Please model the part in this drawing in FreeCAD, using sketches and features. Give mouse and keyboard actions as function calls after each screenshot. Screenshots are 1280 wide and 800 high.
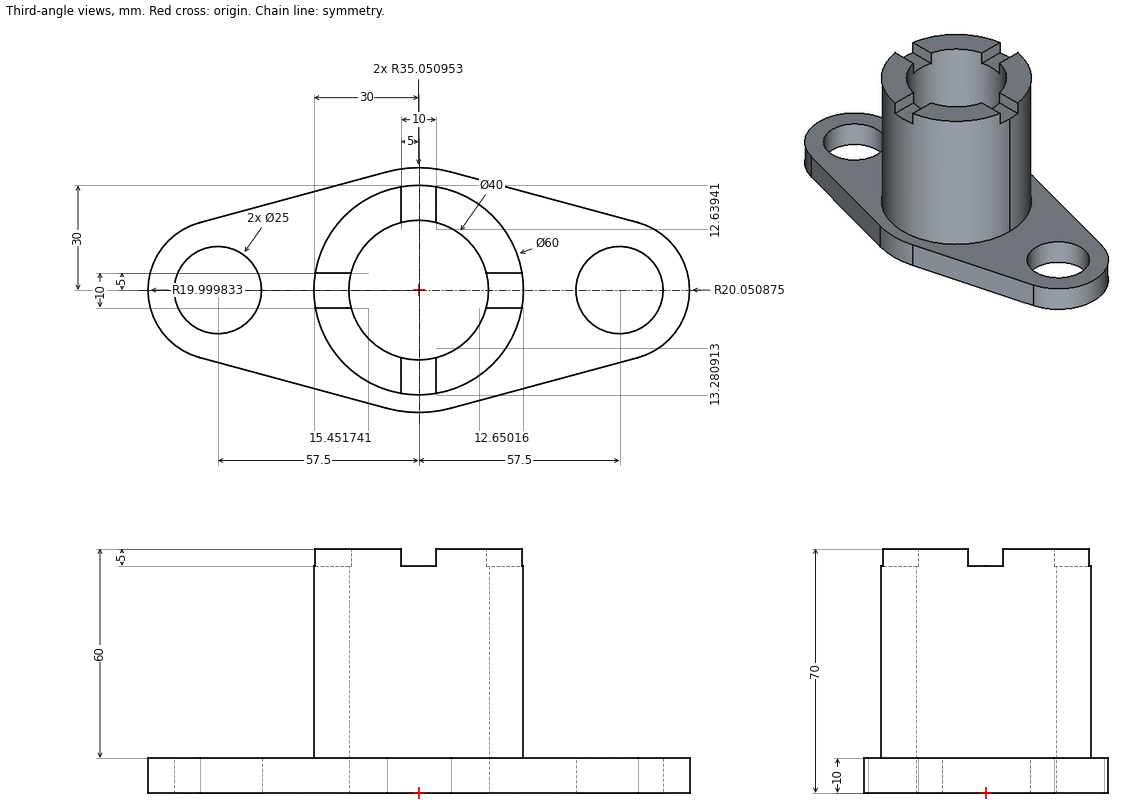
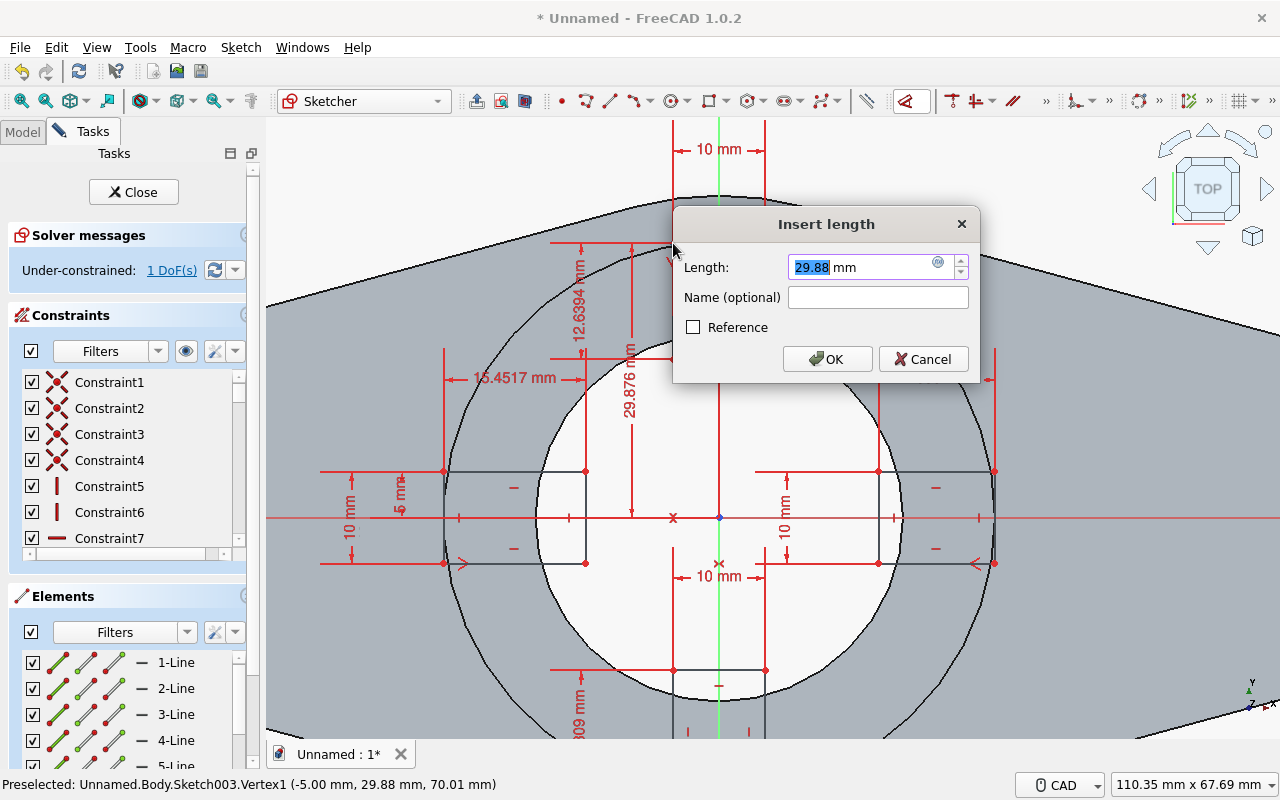
text(30)
key(Return)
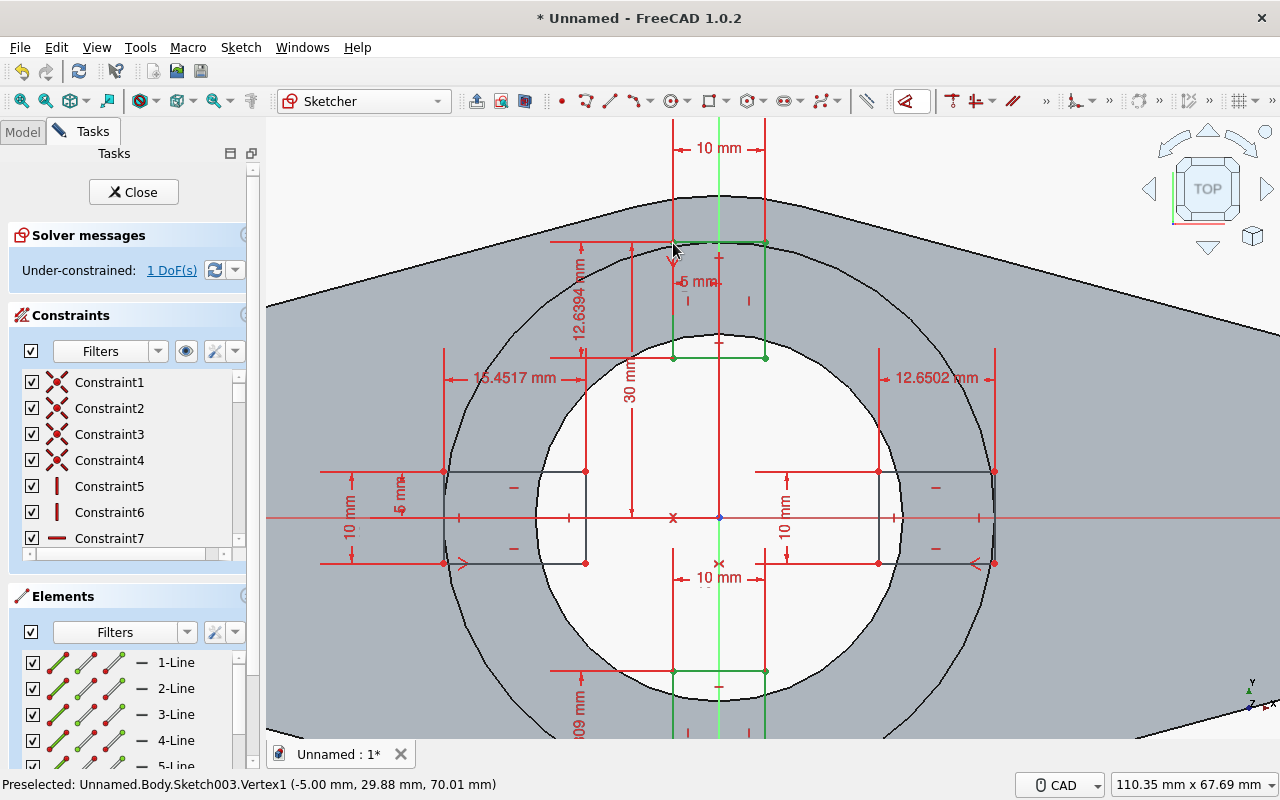
click(444, 472)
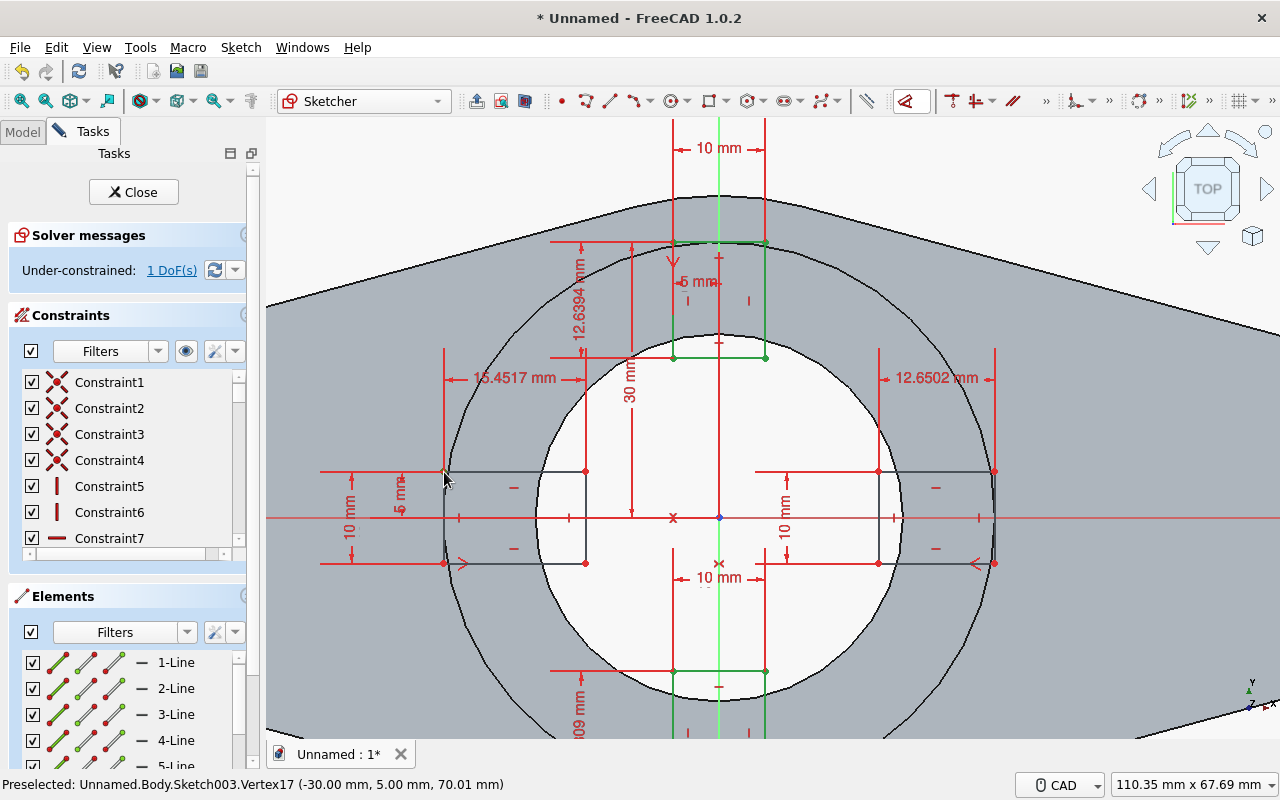
key(l)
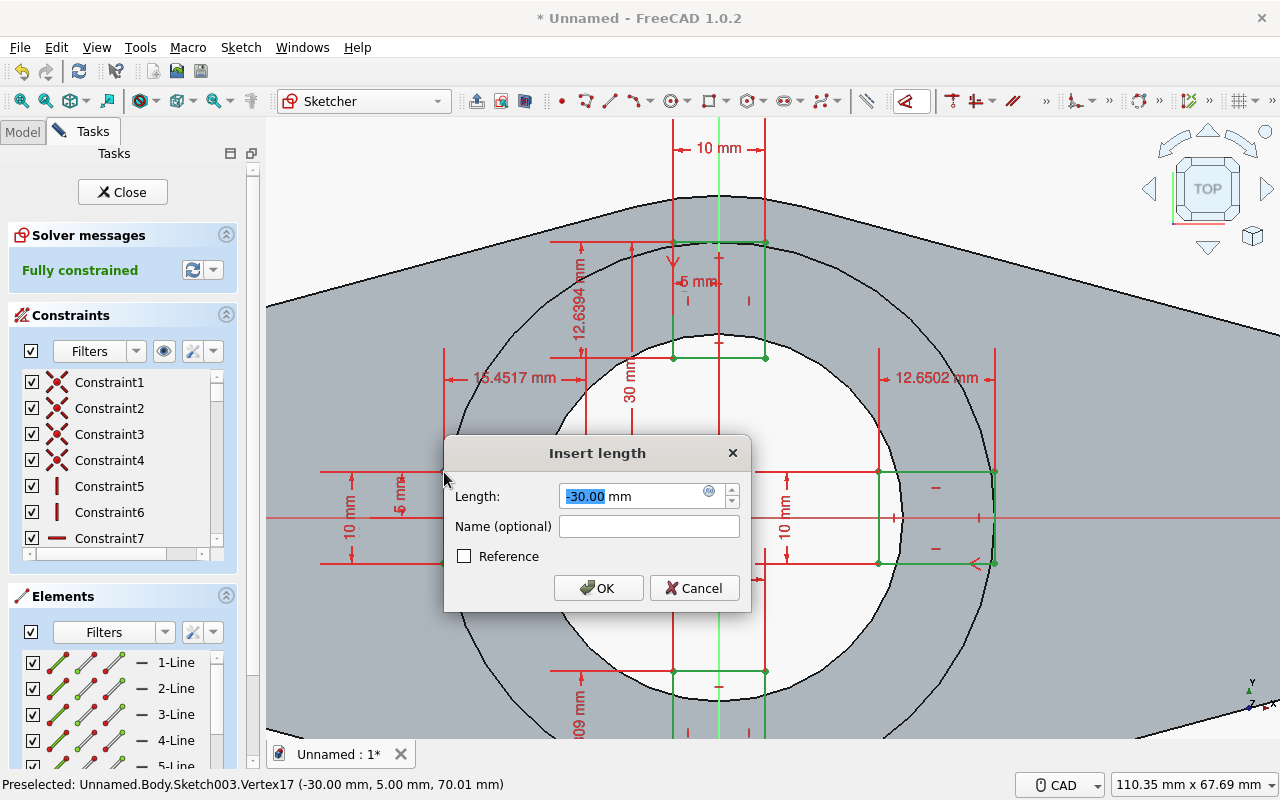
text(-30)
key(Return)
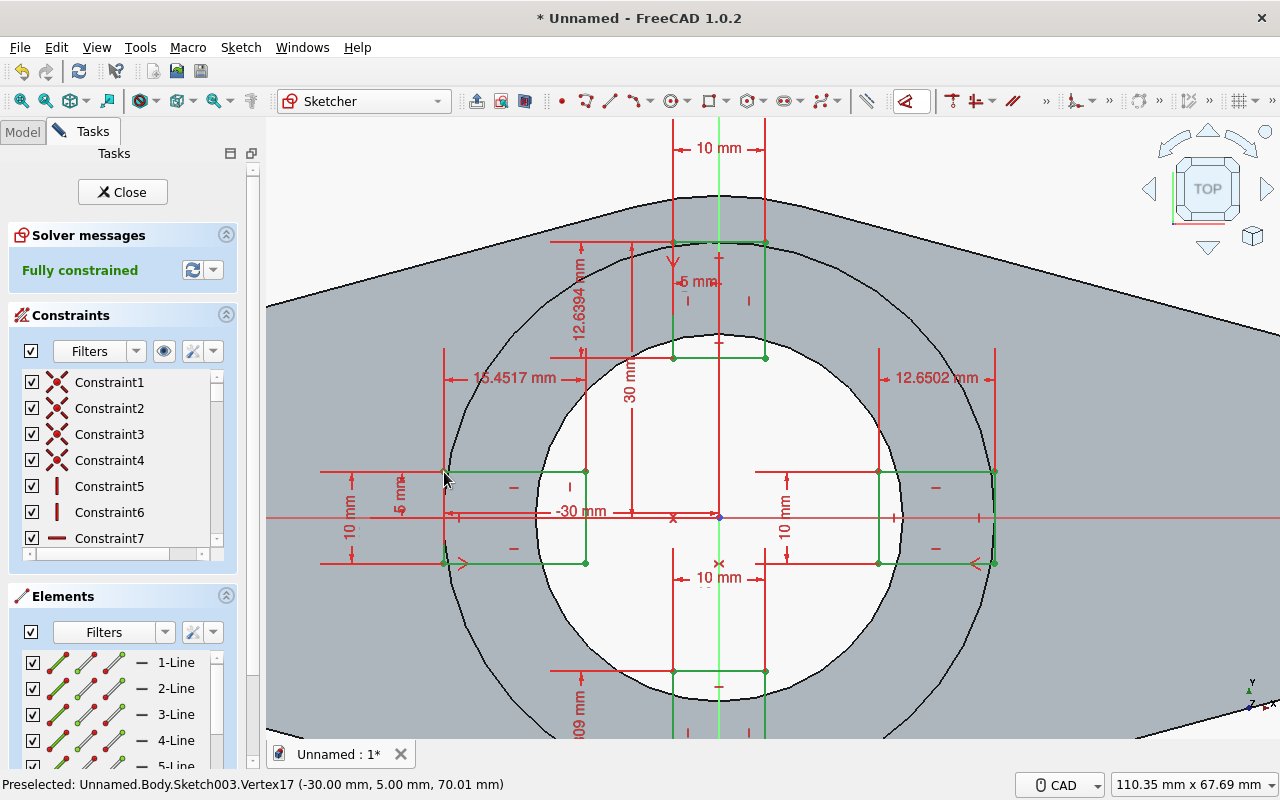
click(123, 192)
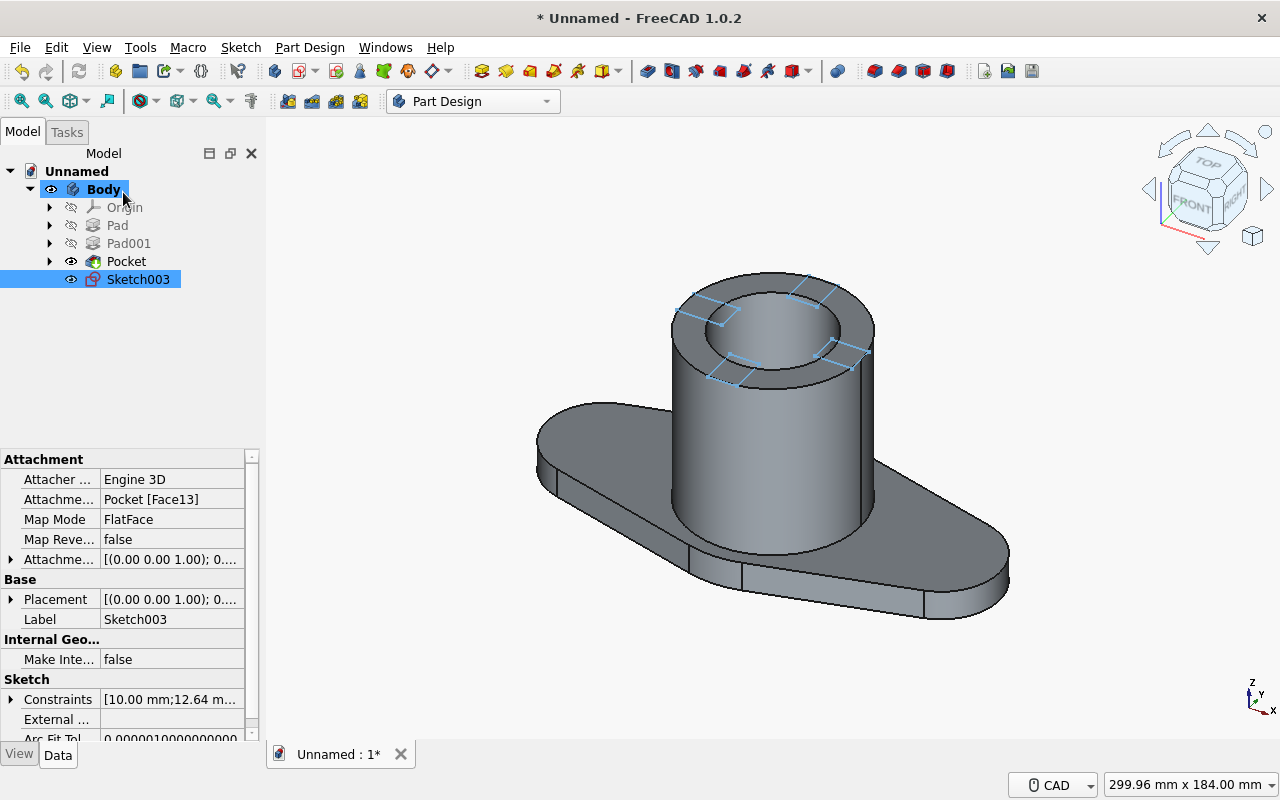
click(648, 72)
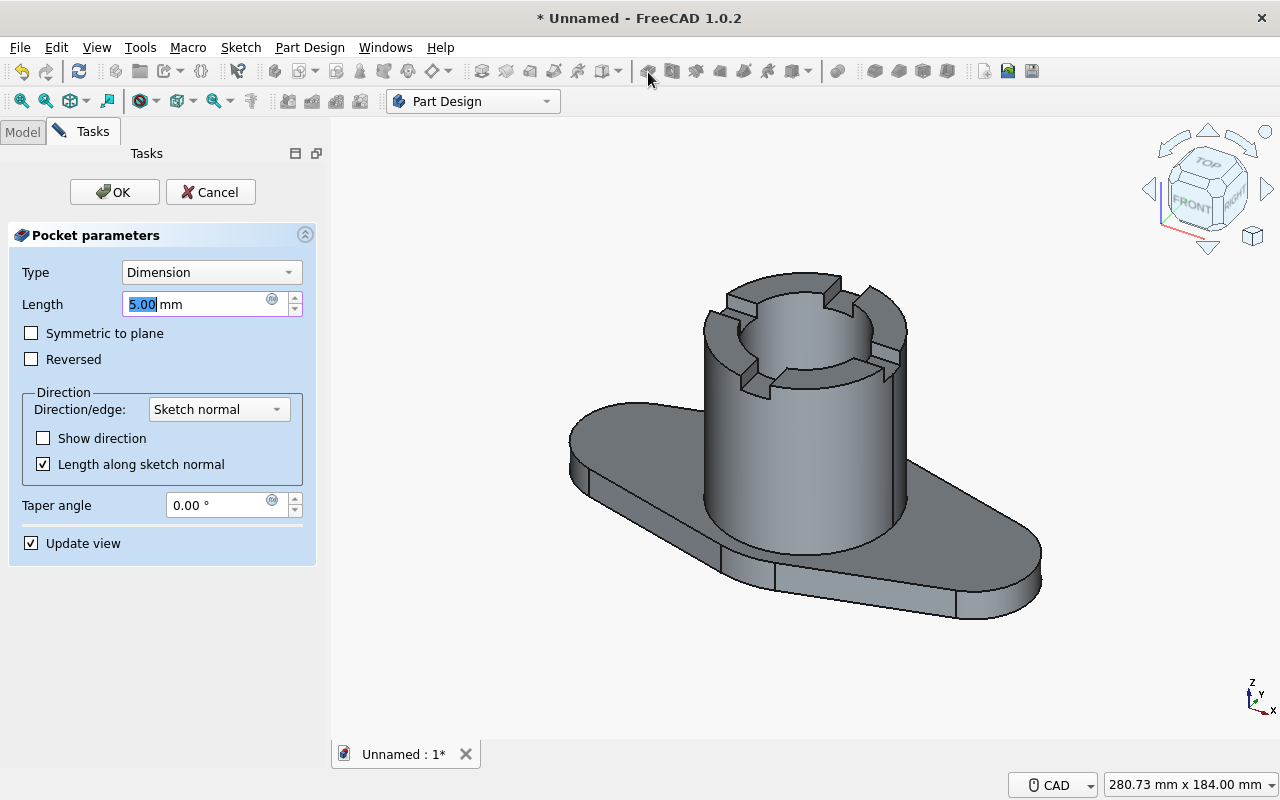
text(5)
key(Tab)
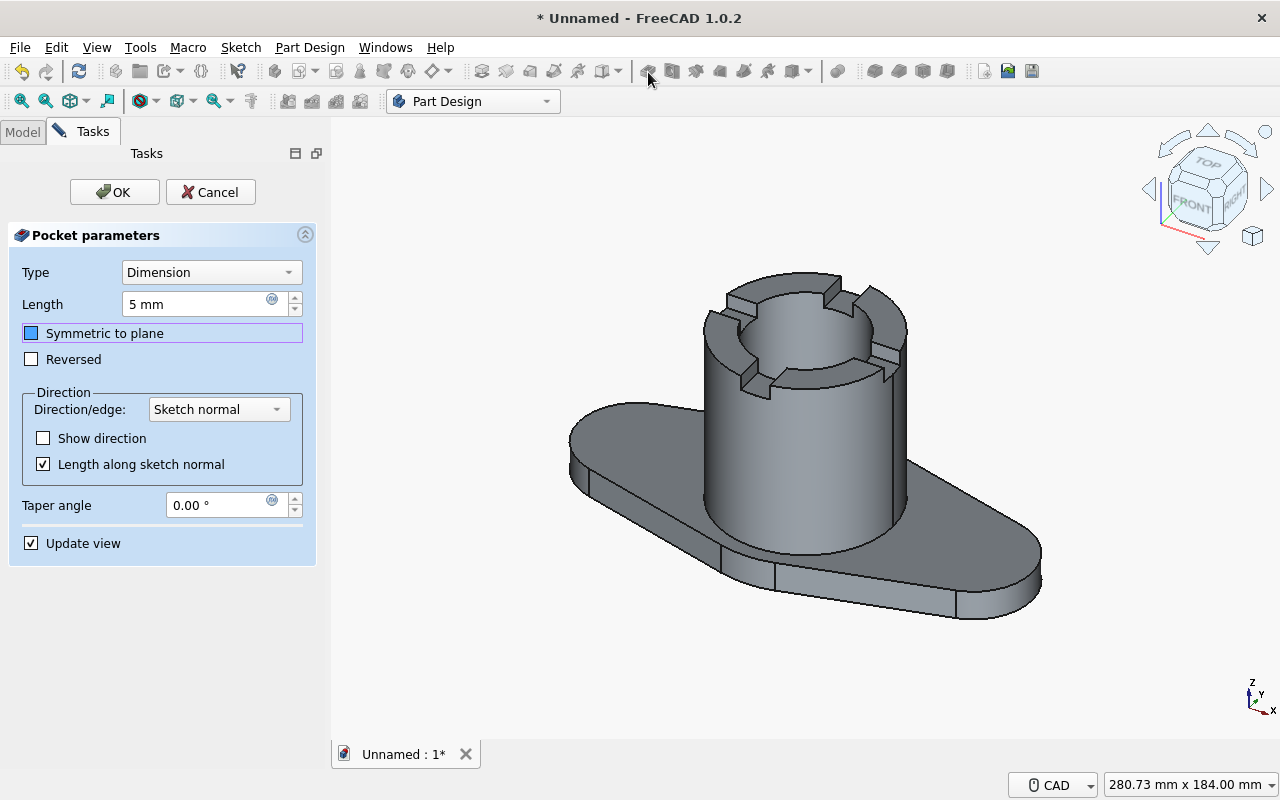
click(115, 192)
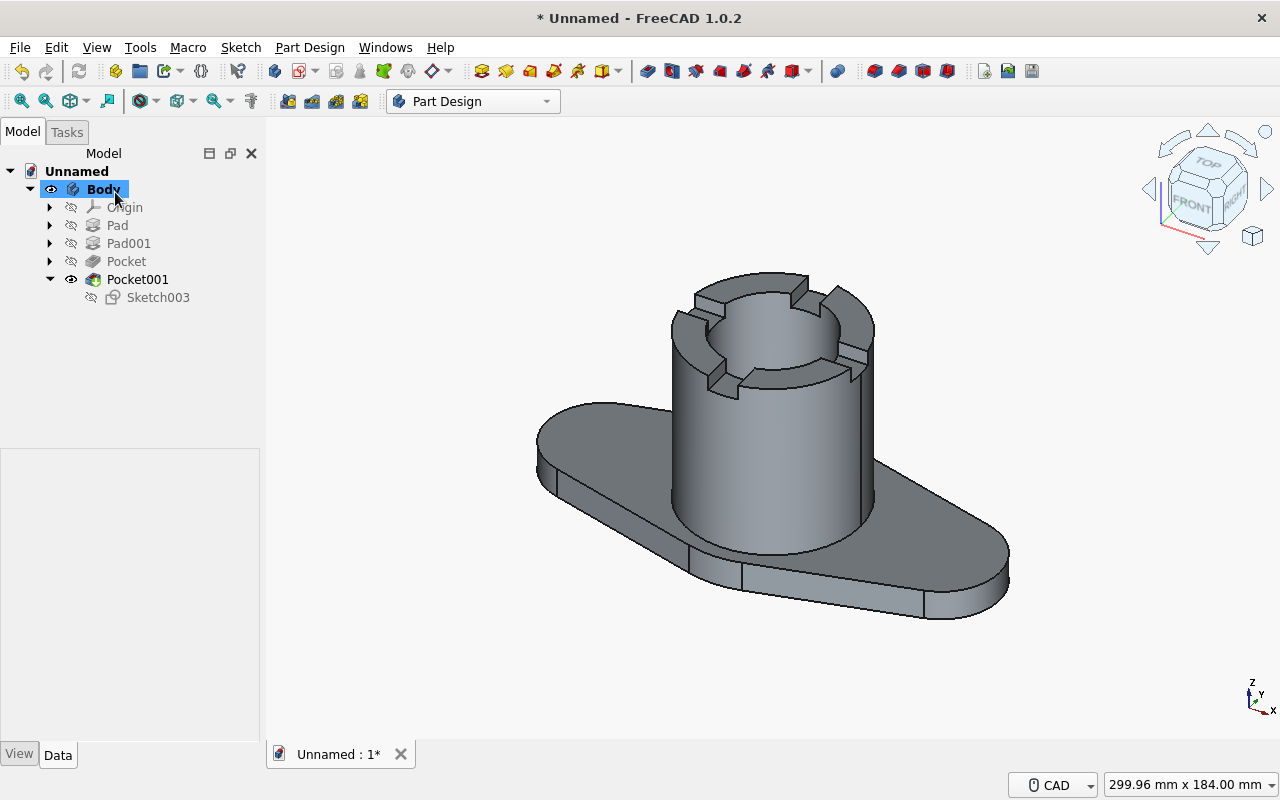
click(903, 539)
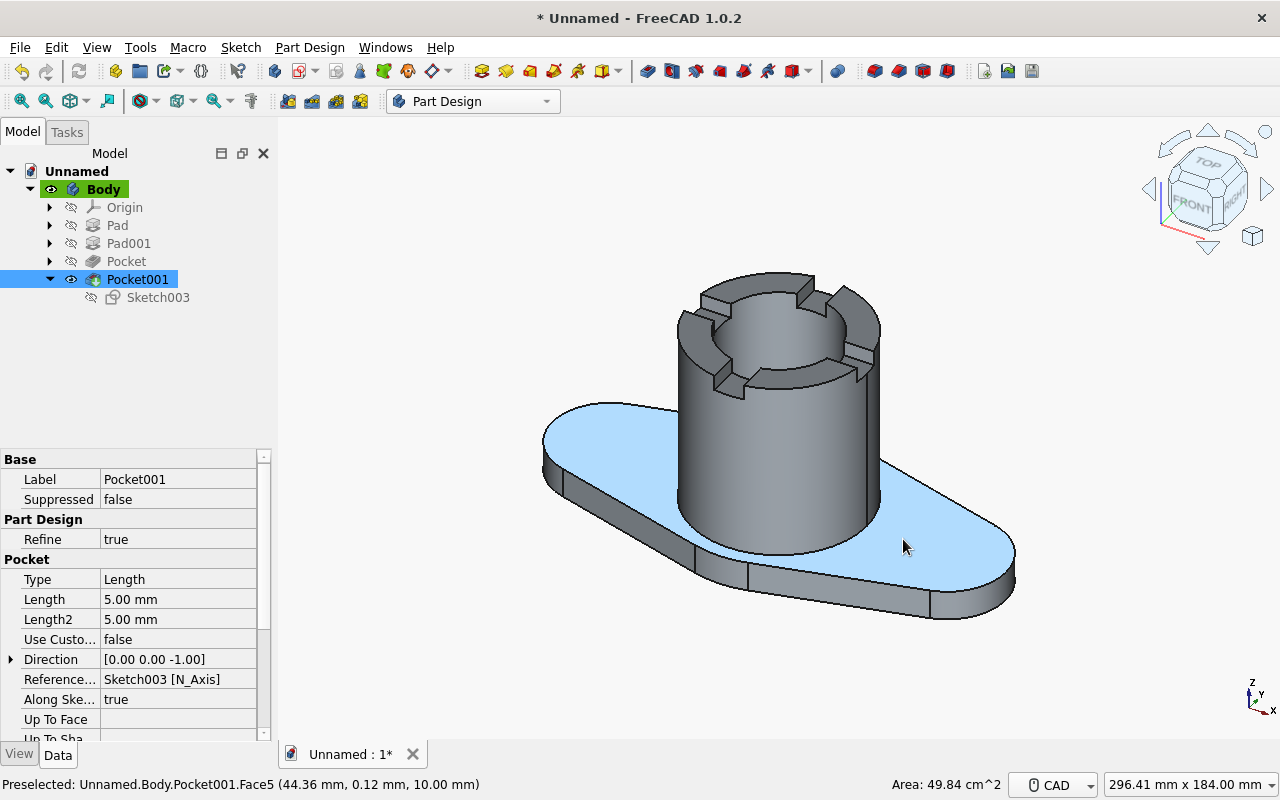
click(300, 72)